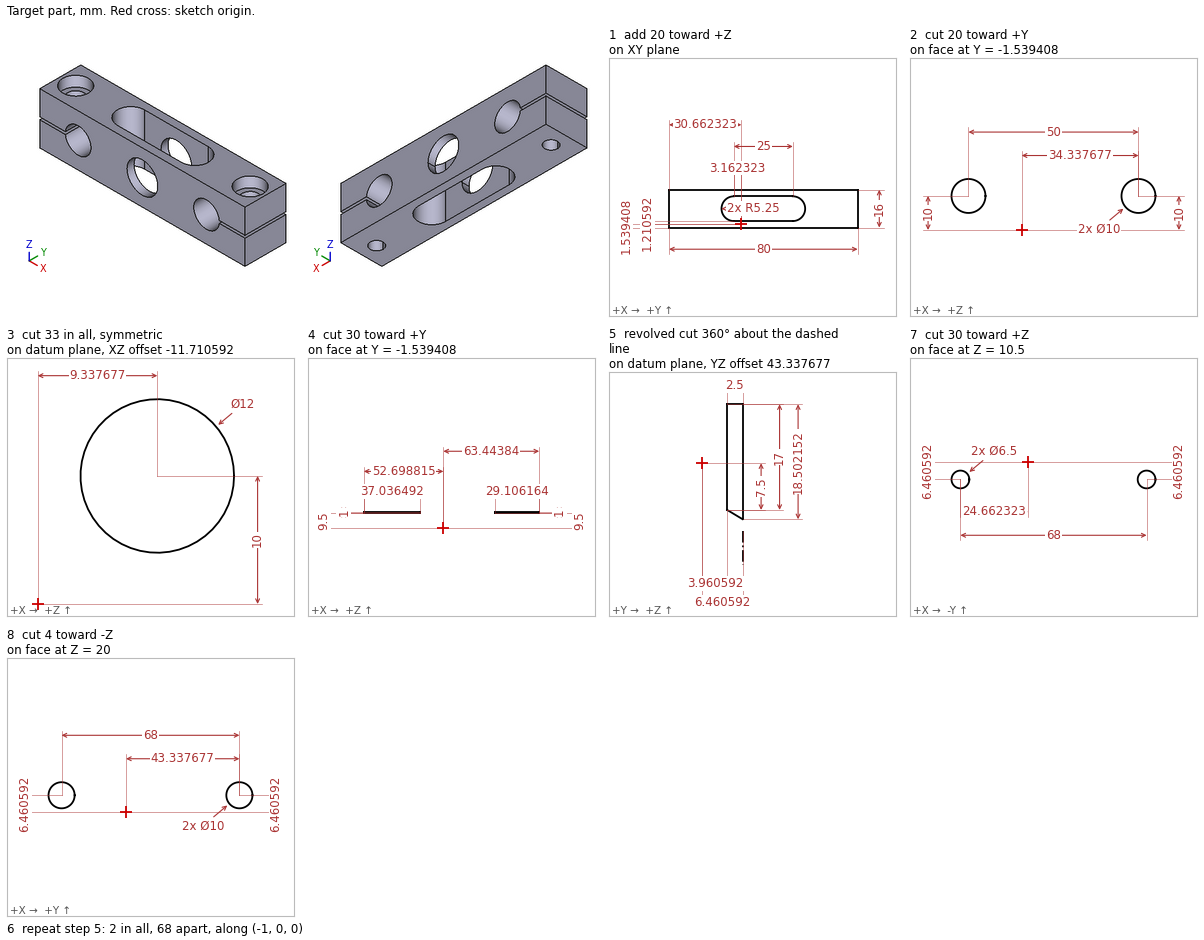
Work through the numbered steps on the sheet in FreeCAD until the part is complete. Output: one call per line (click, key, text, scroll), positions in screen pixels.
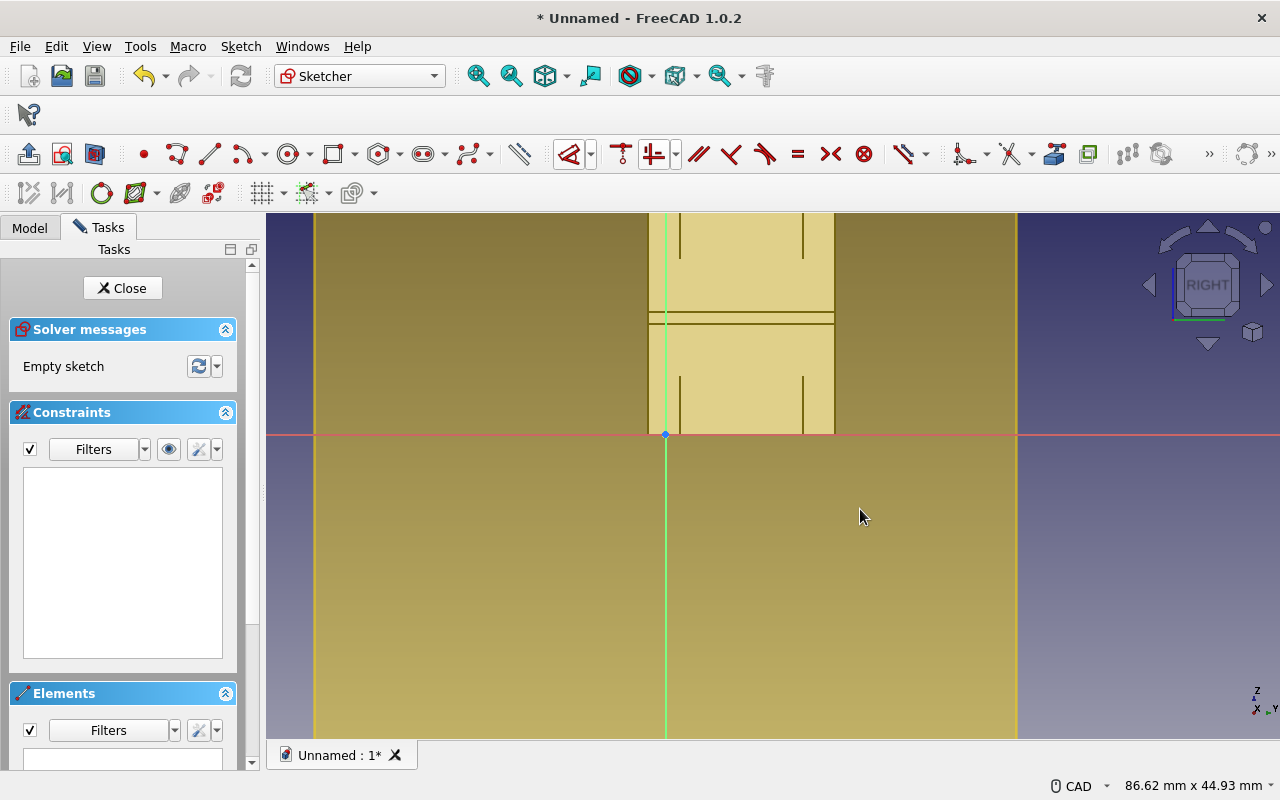
click(177, 154)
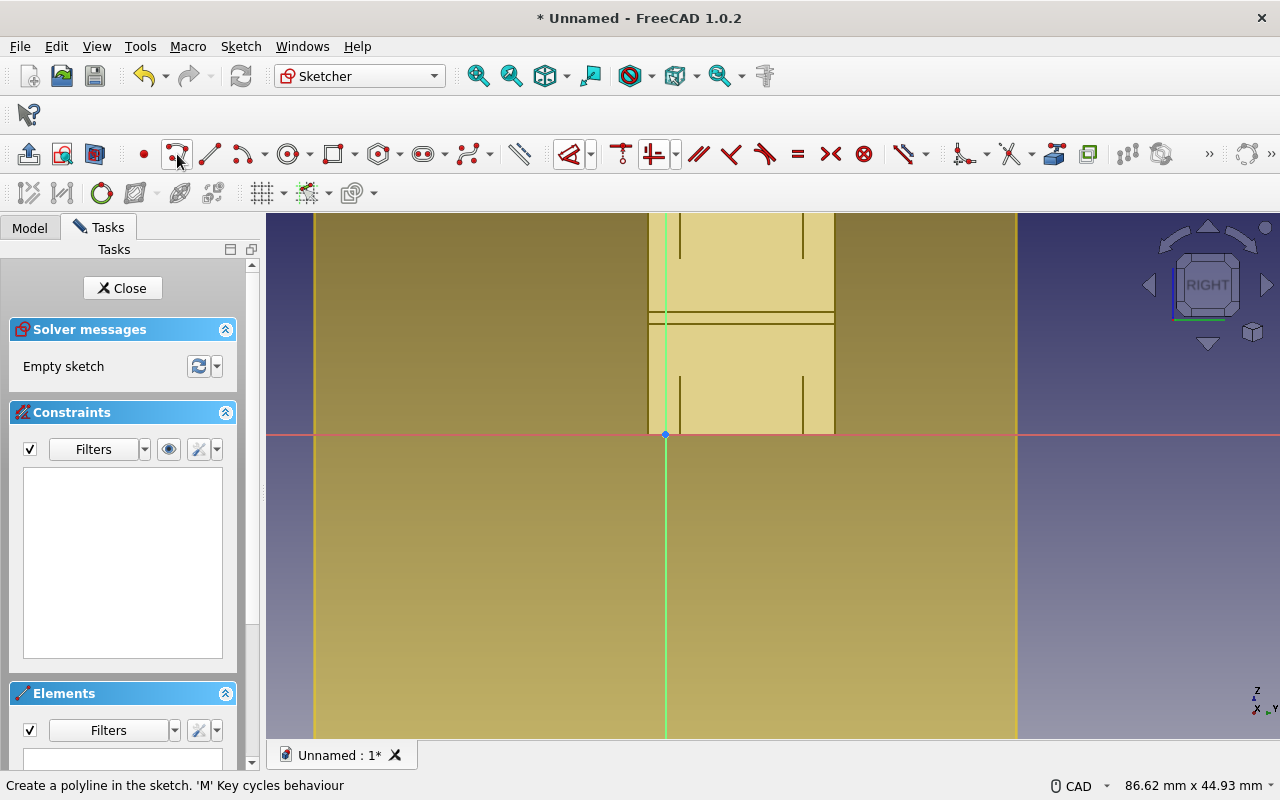
click(712, 523)
click(741, 540)
click(741, 324)
click(712, 324)
click(712, 524)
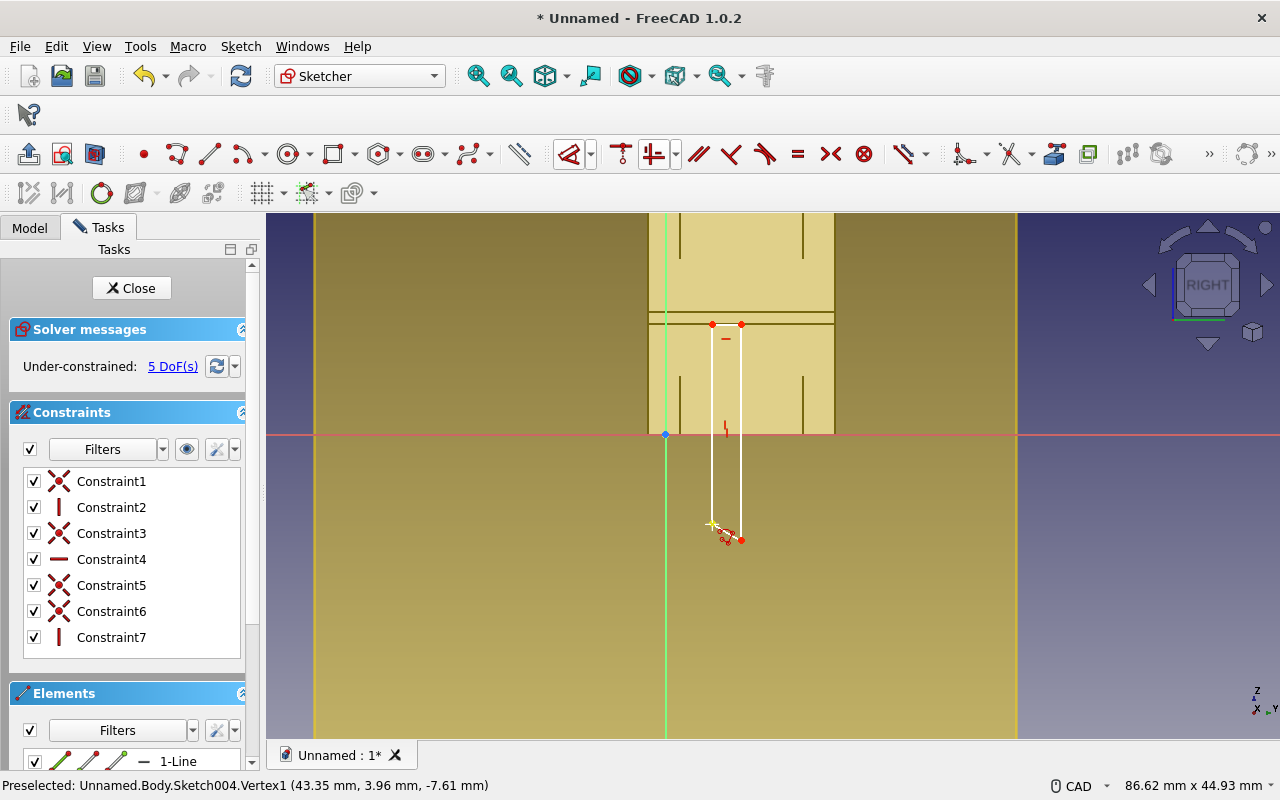
click(210, 154)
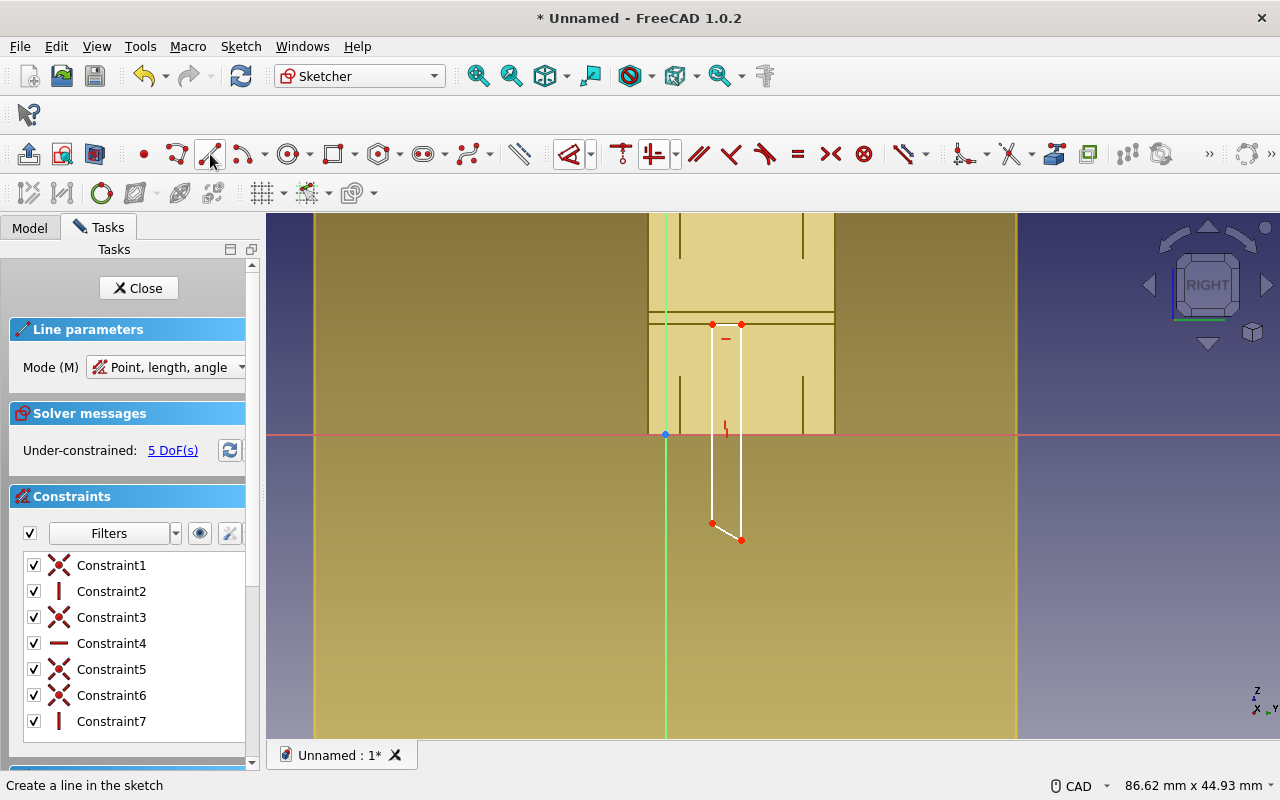
click(741, 562)
click(741, 627)
key(Escape)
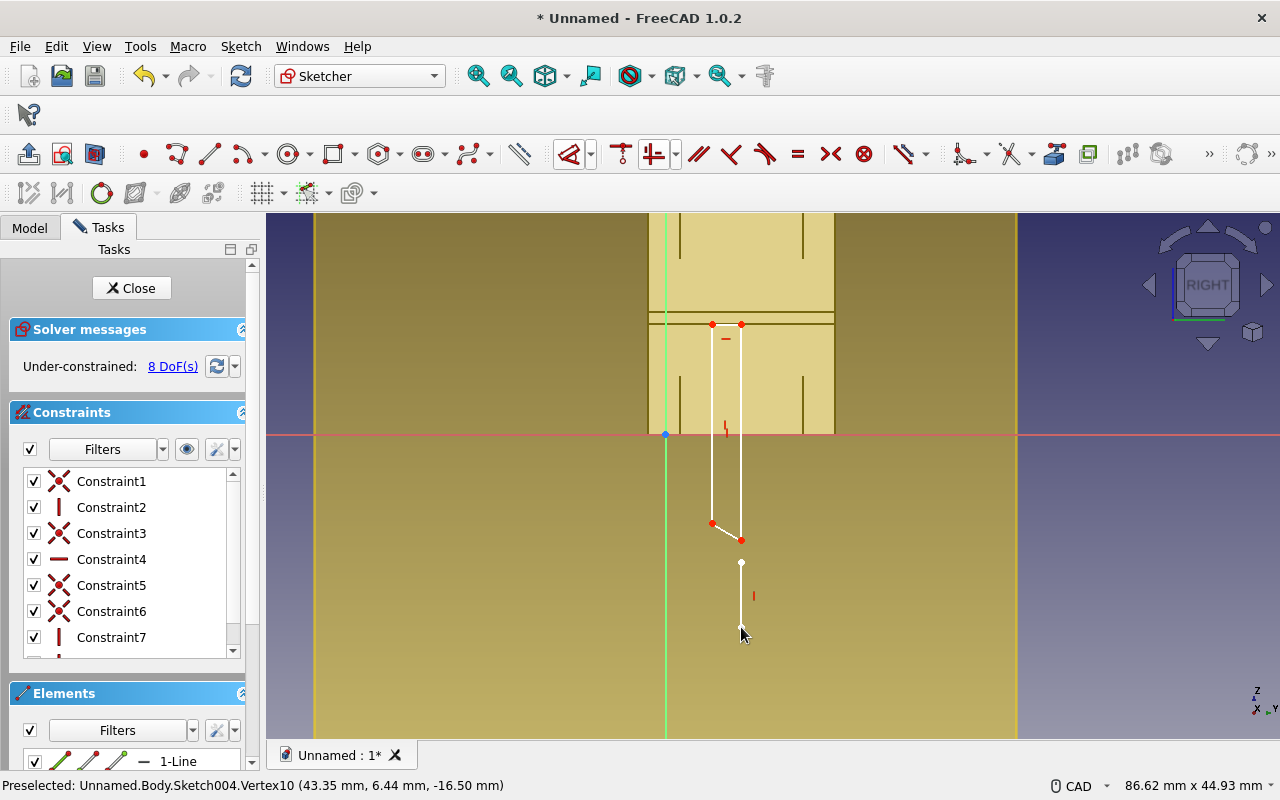
click(741, 583)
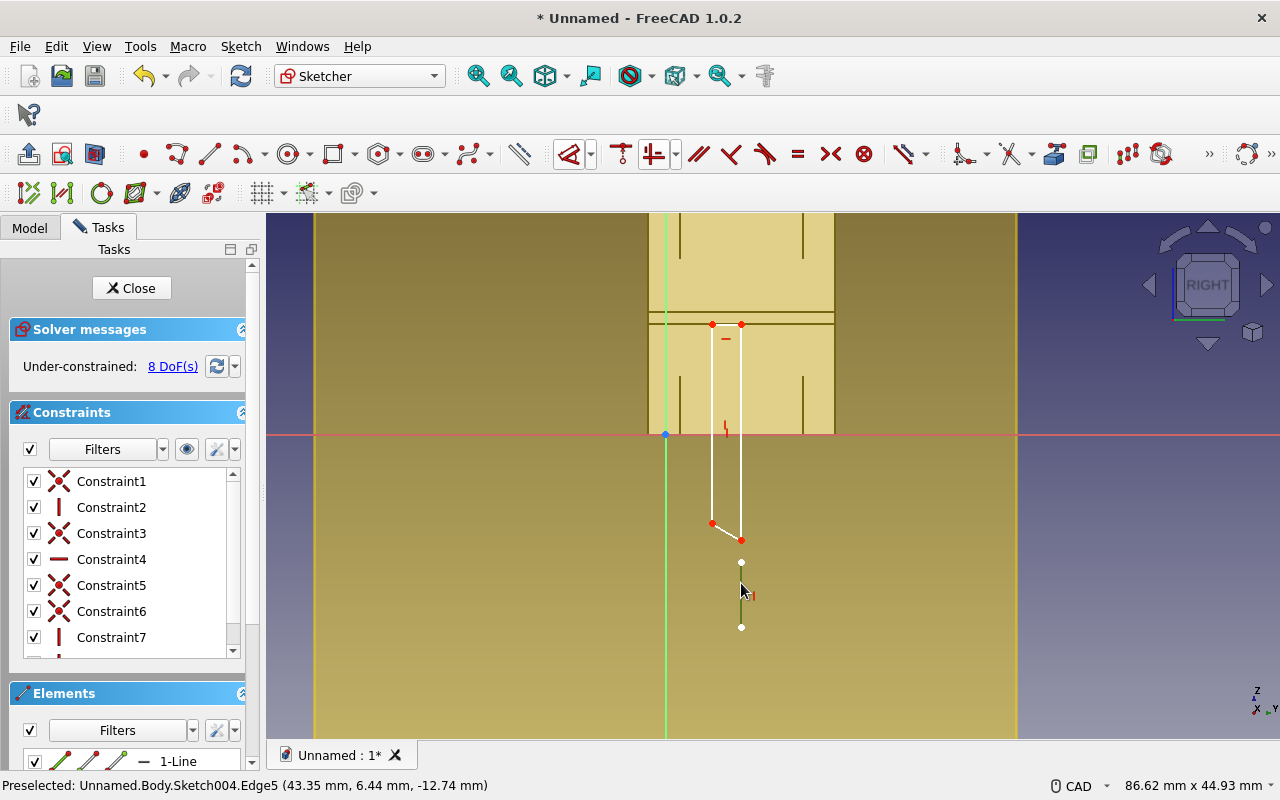
click(520, 154)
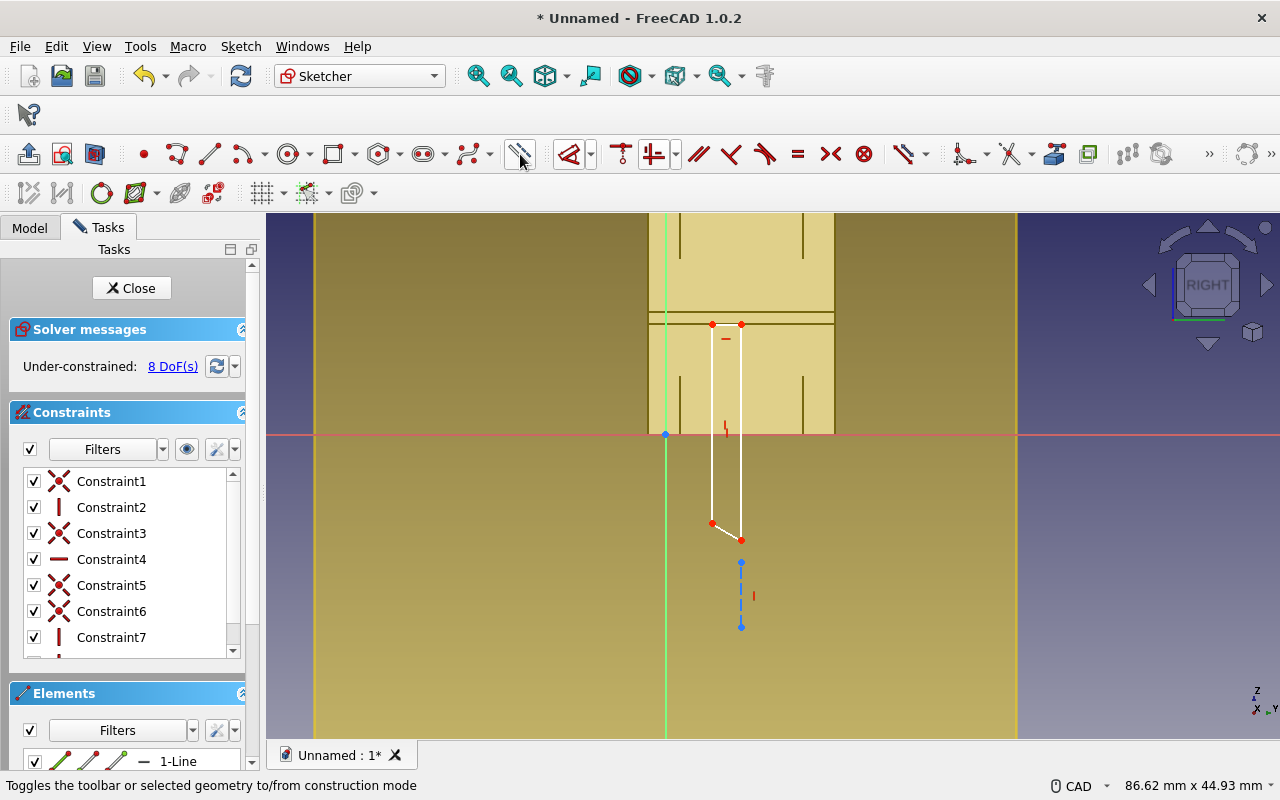
click(712, 385)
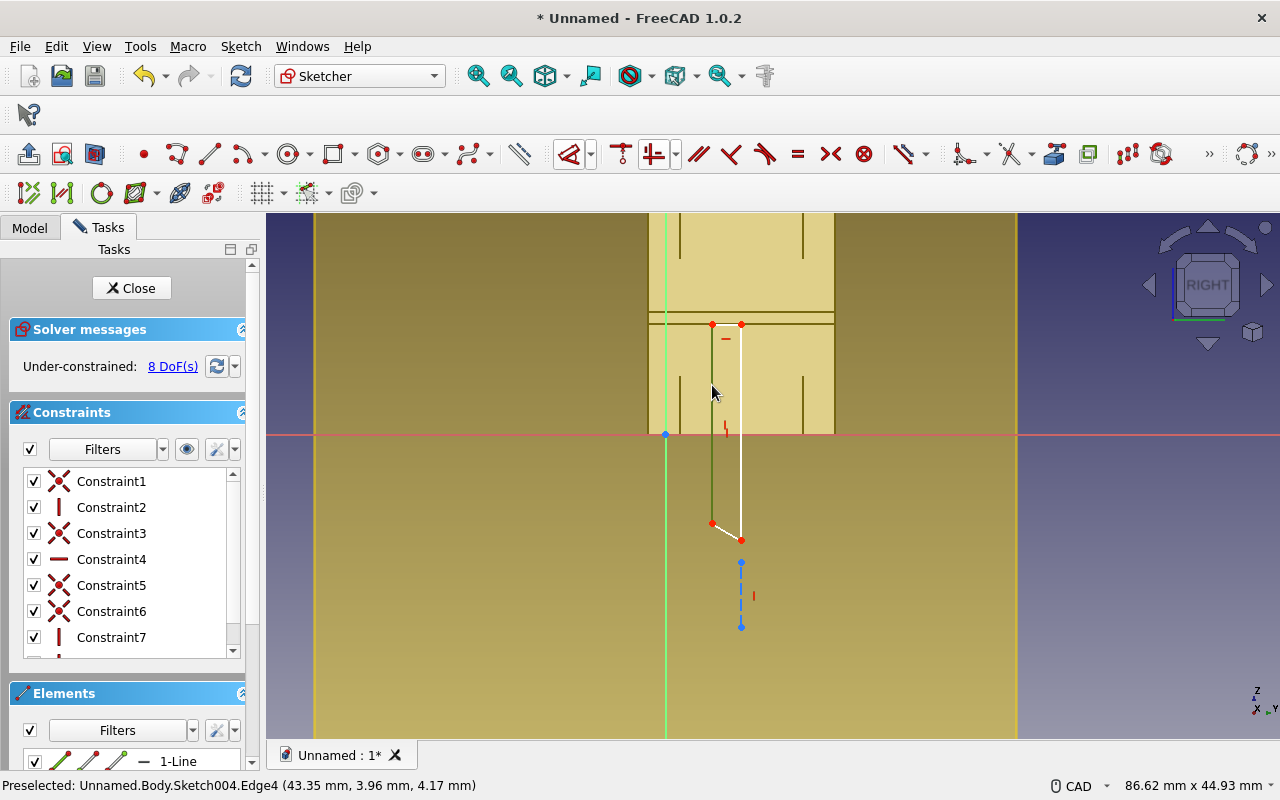
key(i)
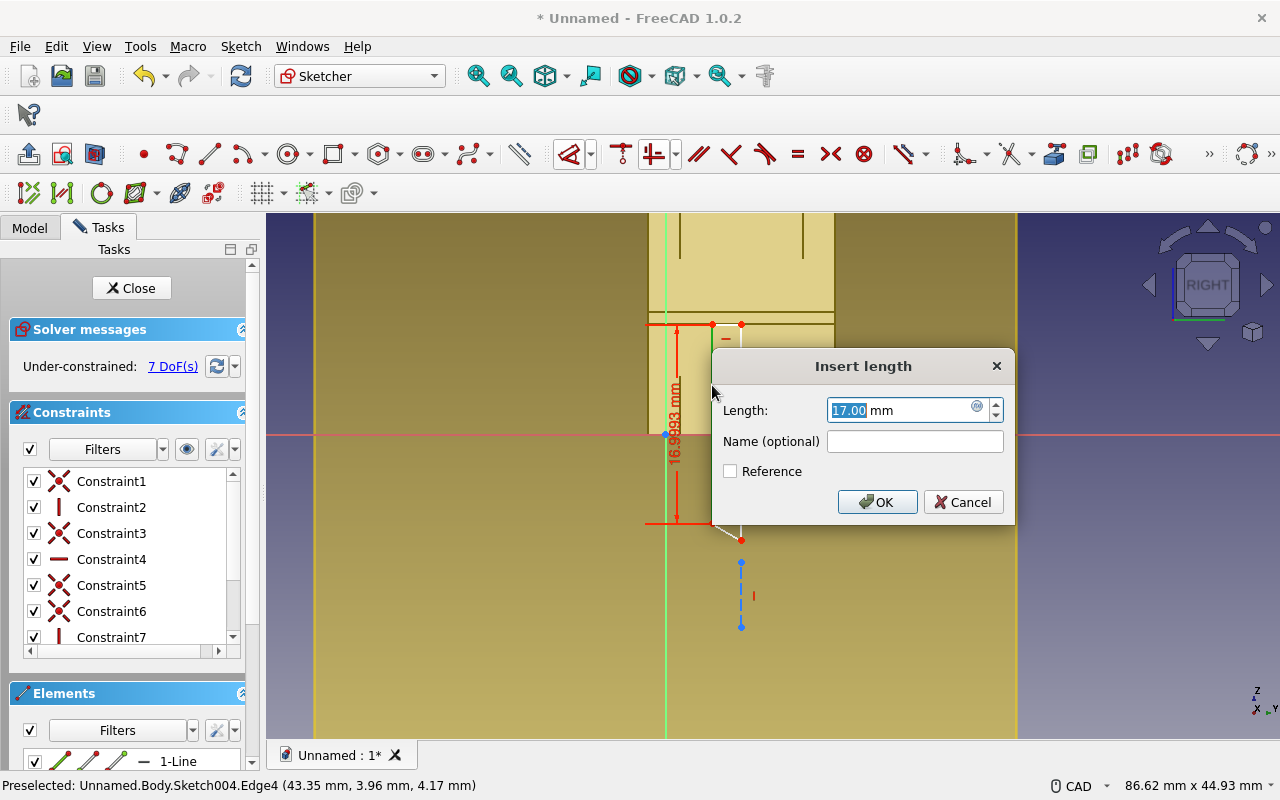
text(17)
key(Return)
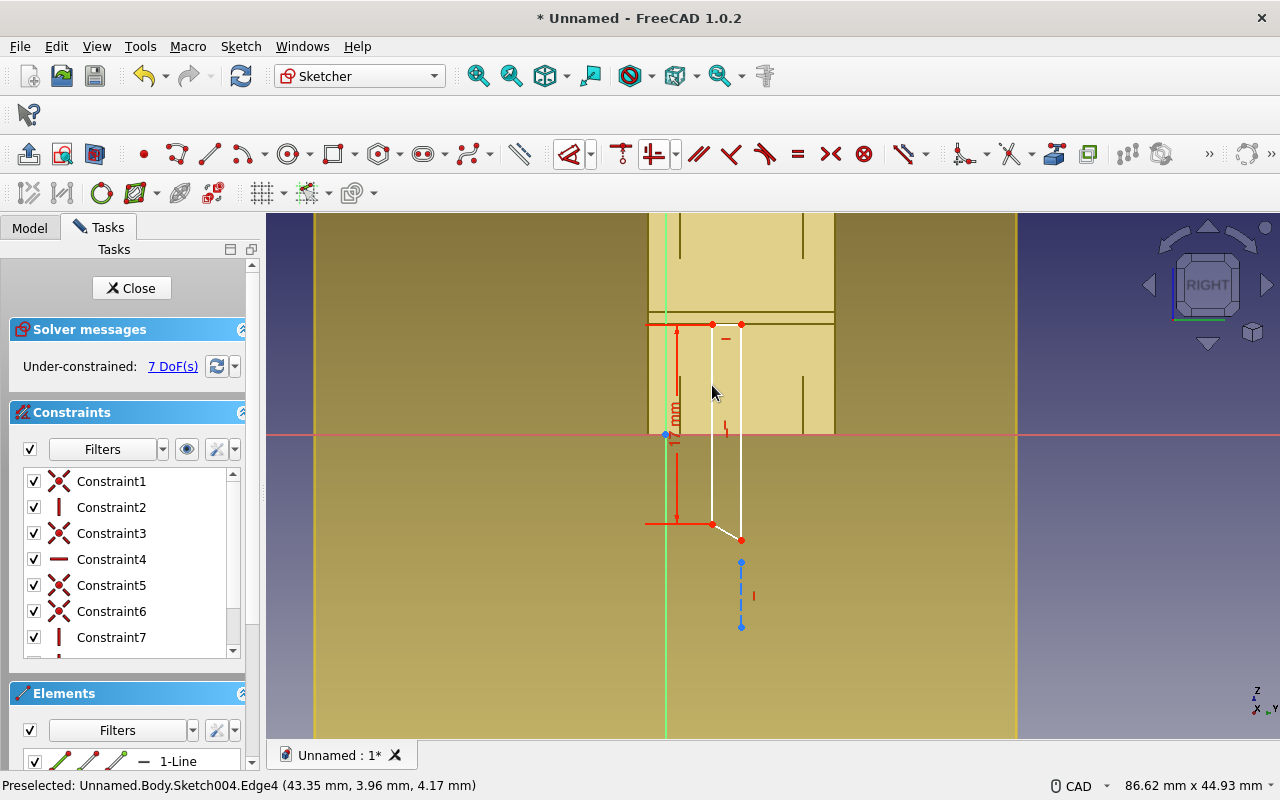
scroll(729, 325, up, 2)